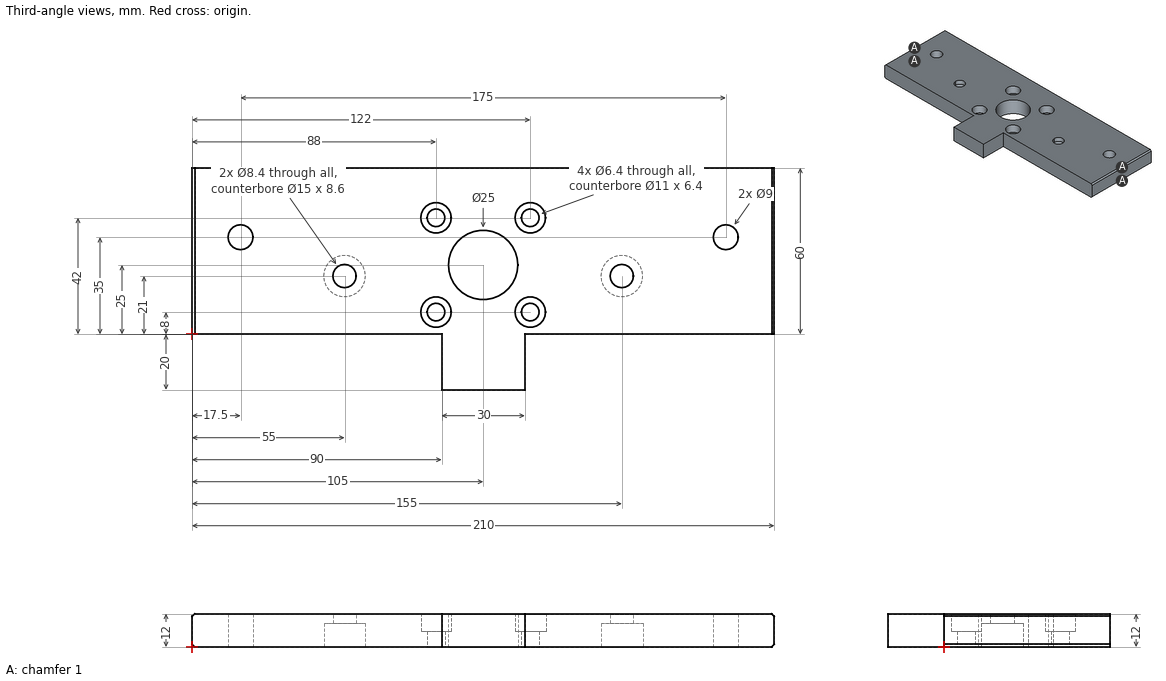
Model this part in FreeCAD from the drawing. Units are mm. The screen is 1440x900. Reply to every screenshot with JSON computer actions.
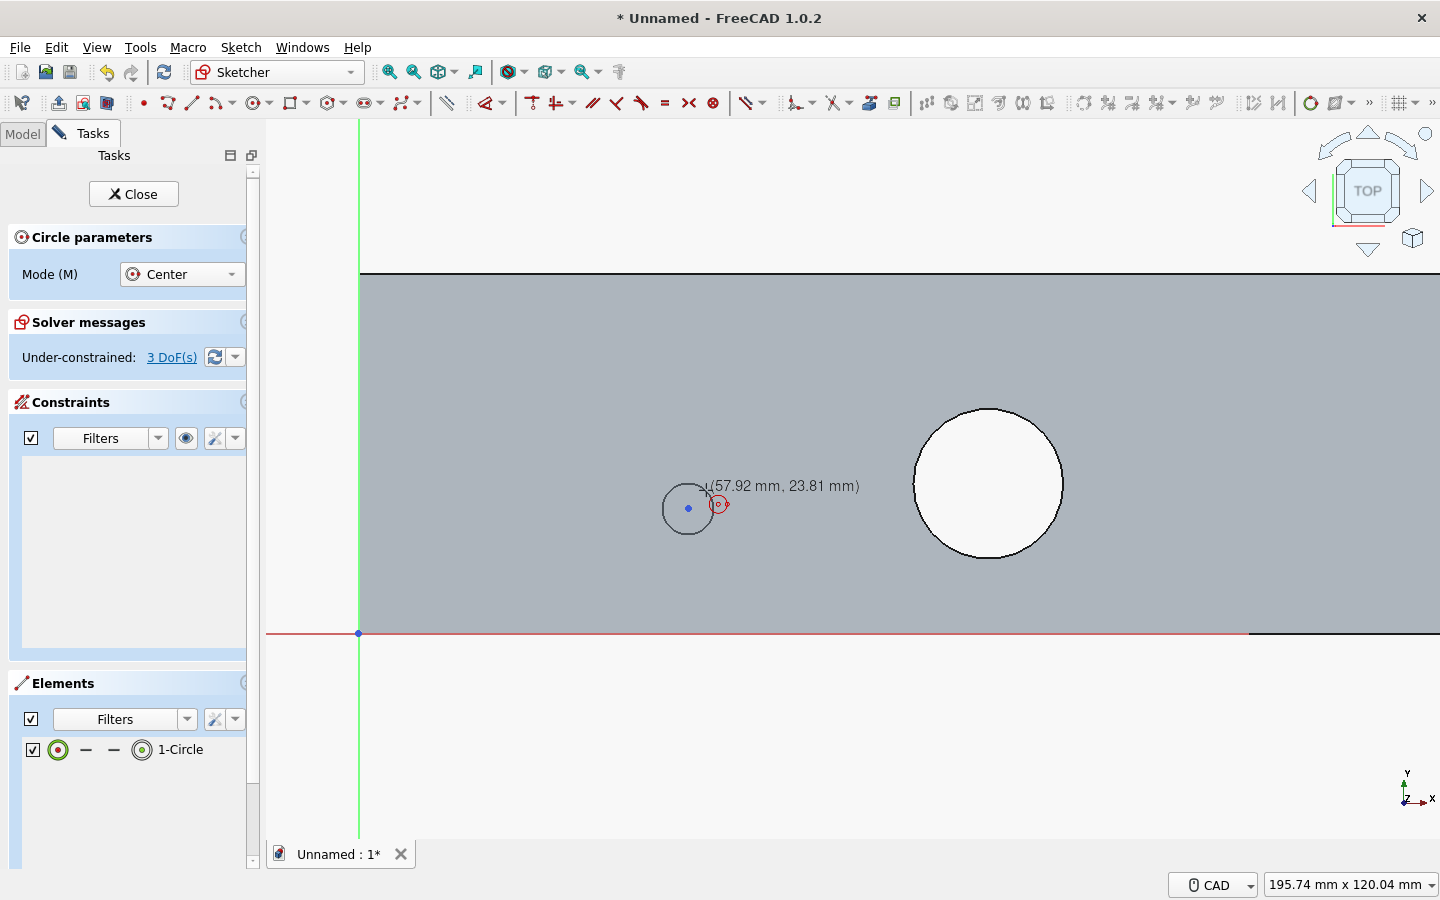
{"action": "scroll", "coordinate": [680, 318], "scroll_direction": "down", "scroll_amount": 2}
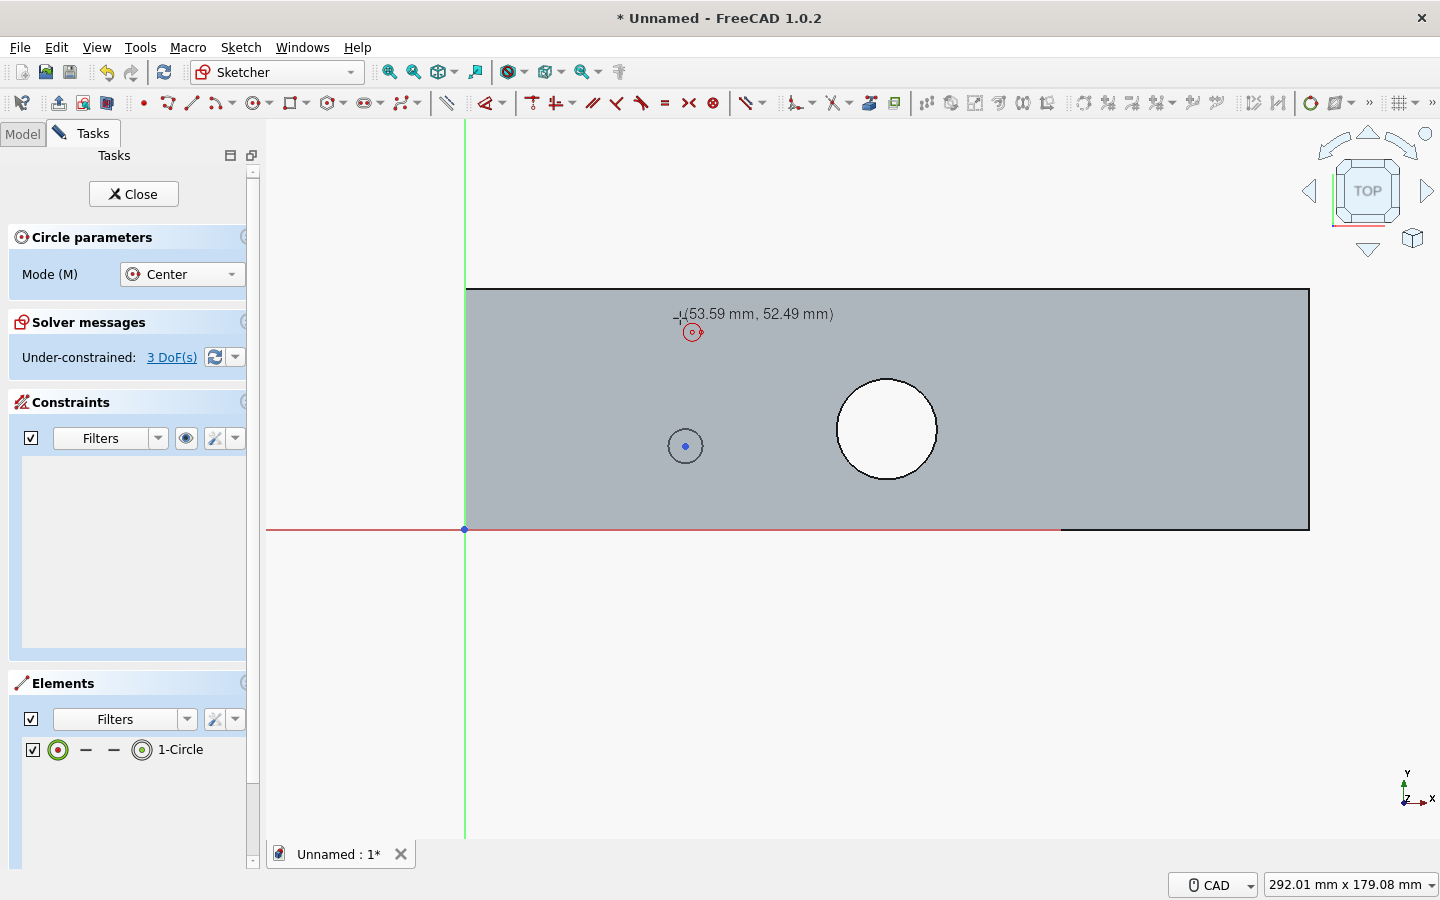
{"action": "scroll", "coordinate": [1088, 445], "scroll_direction": "up", "scroll_amount": 2}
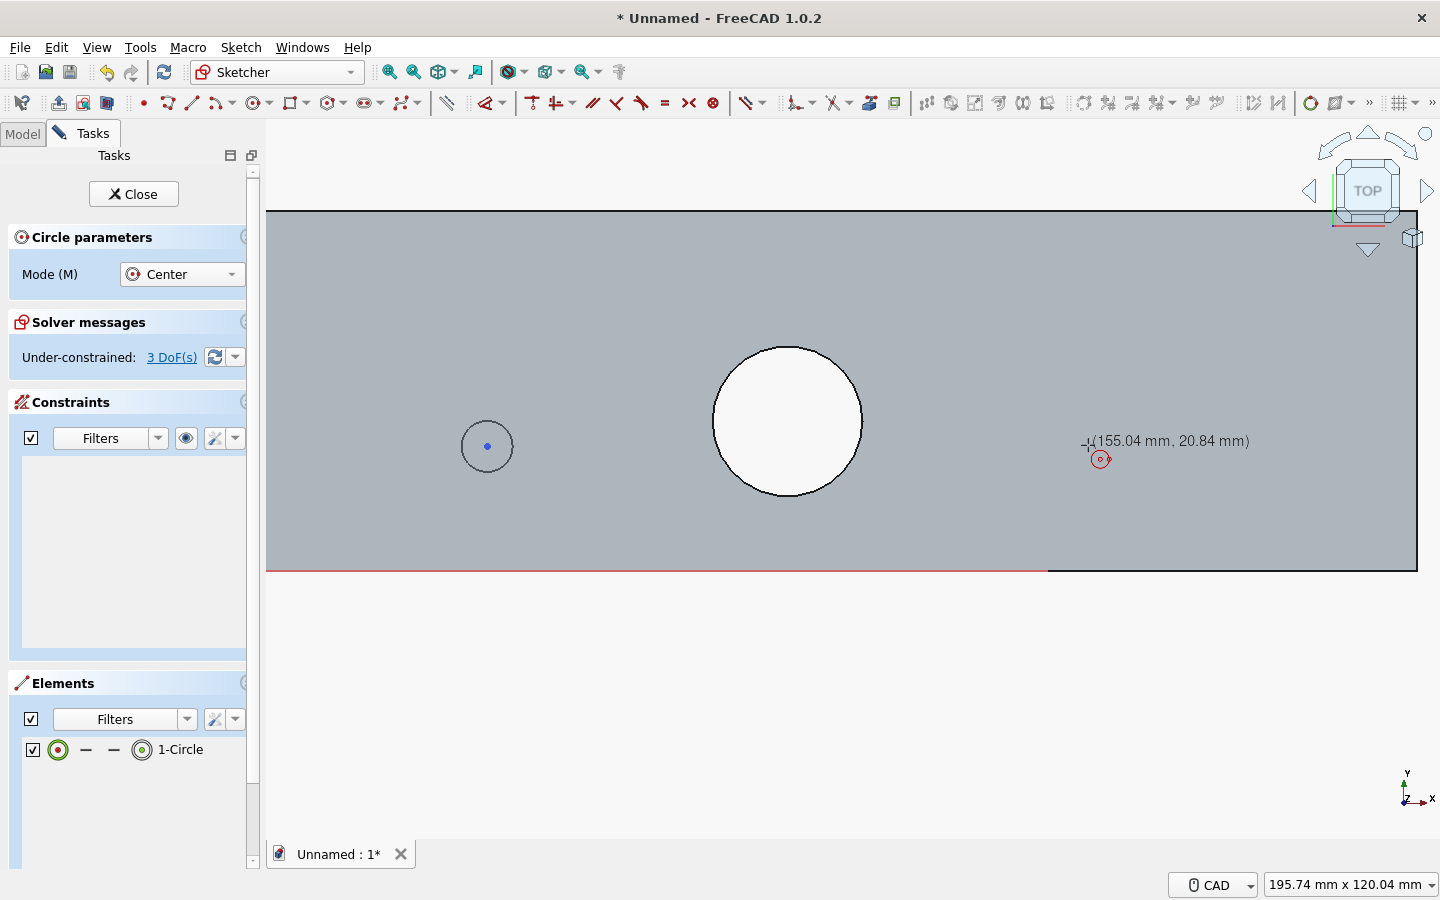
{"action": "left_click", "coordinate": [1087, 445]}
{"action": "left_click", "coordinate": [1105, 428]}
{"action": "key", "text": "Escape"}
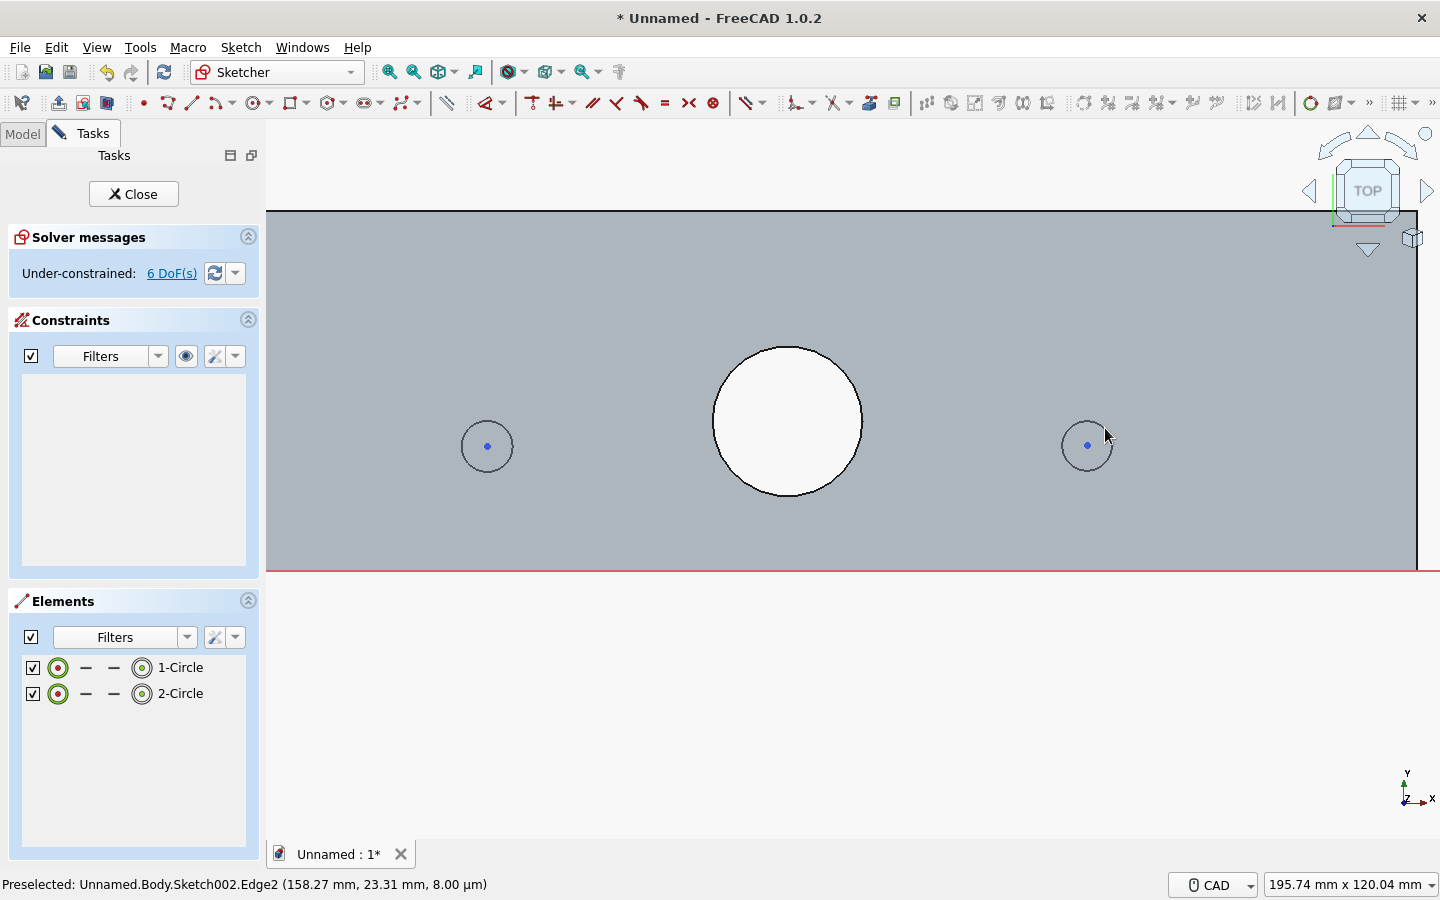
{"action": "left_click", "coordinate": [505, 428]}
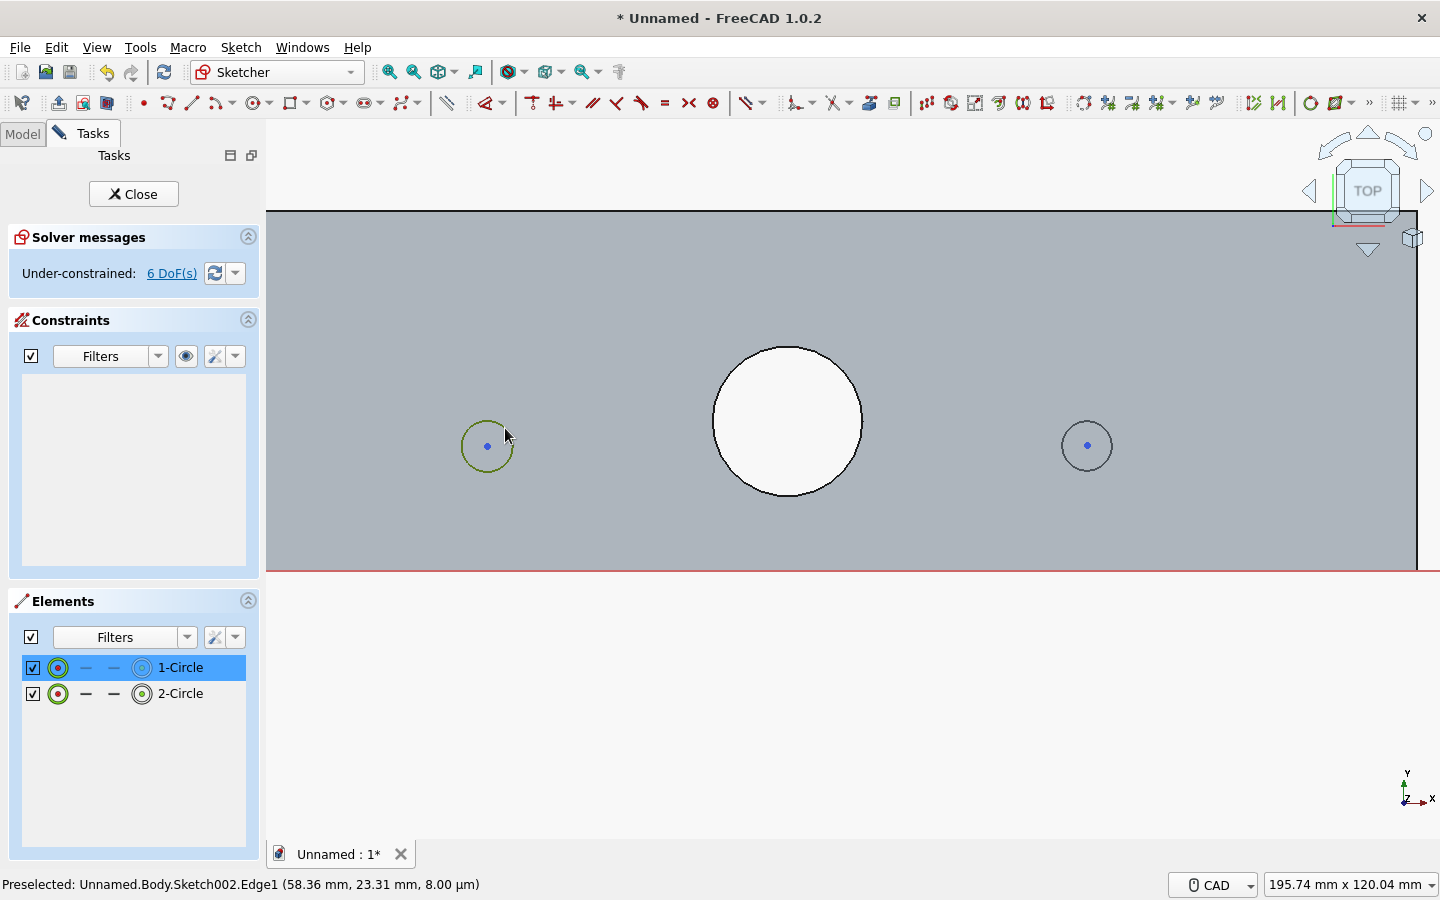
{"action": "left_click", "coordinate": [1104, 428]}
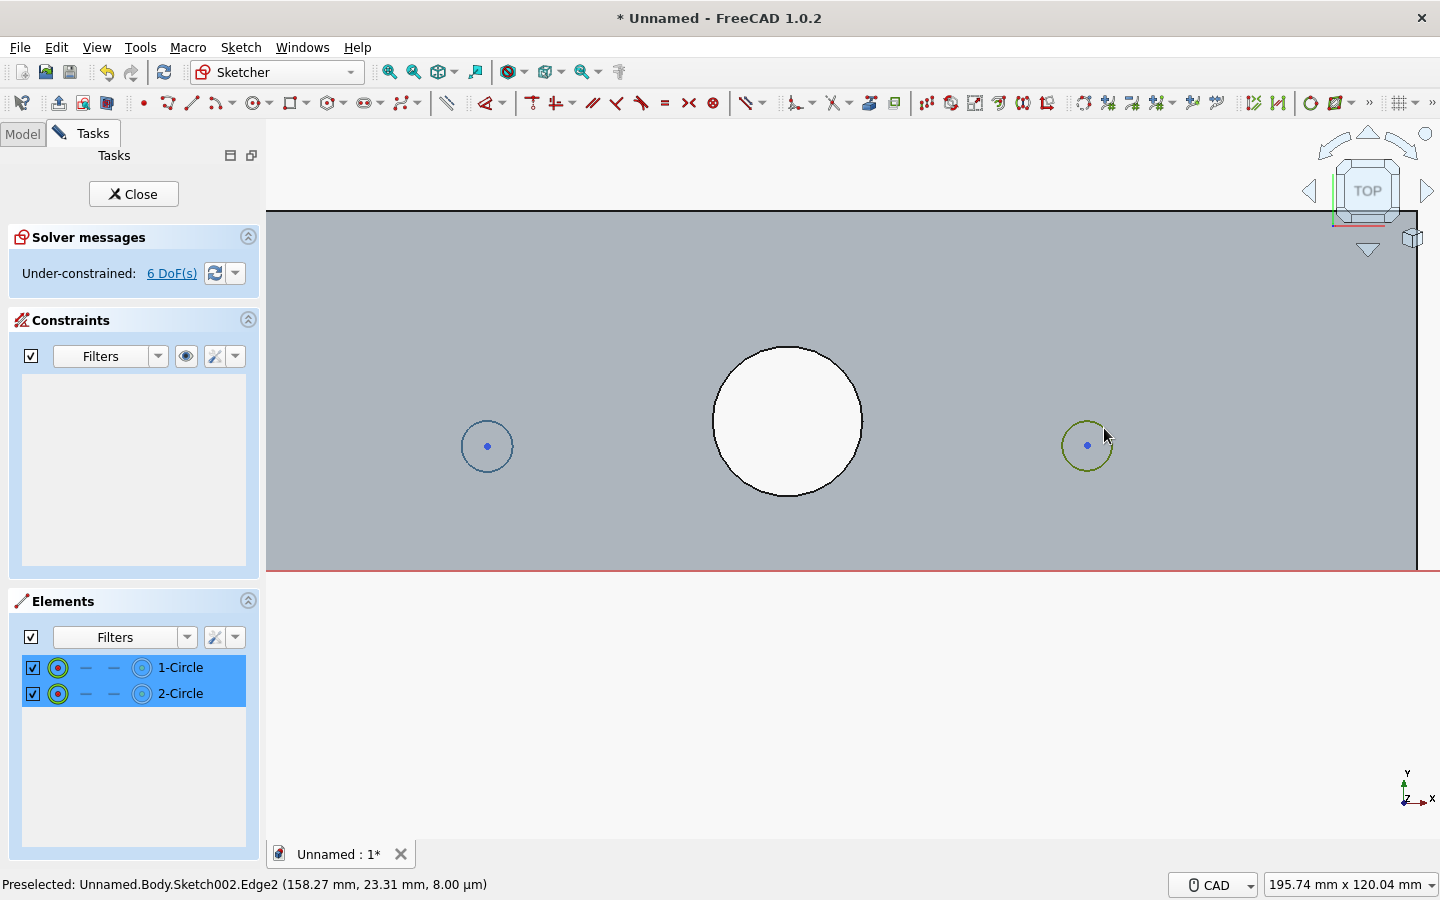
{"action": "left_click", "coordinate": [666, 104]}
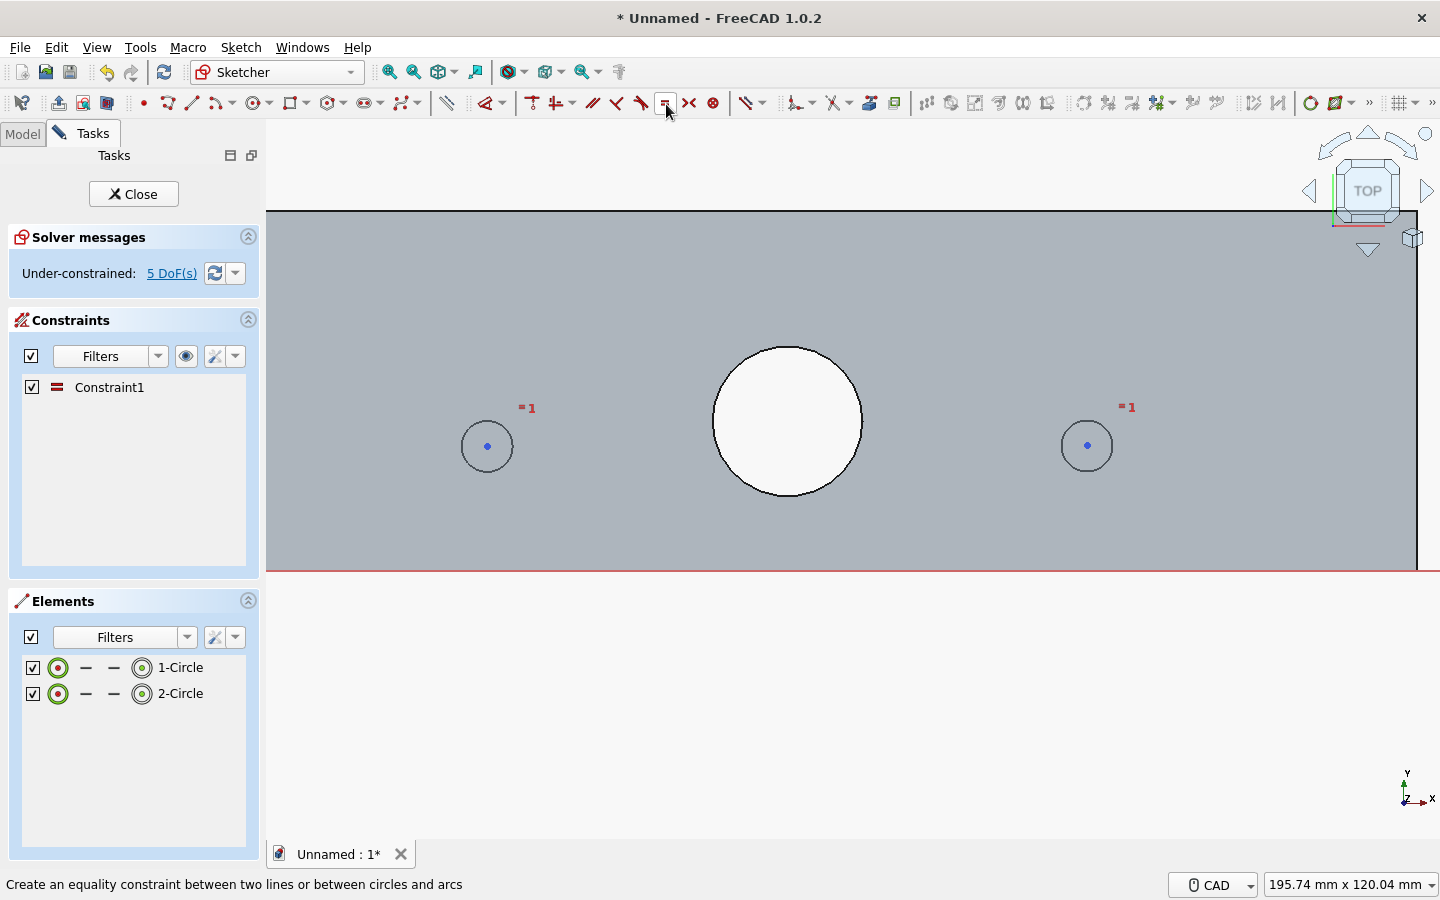
{"action": "left_click", "coordinate": [487, 446]}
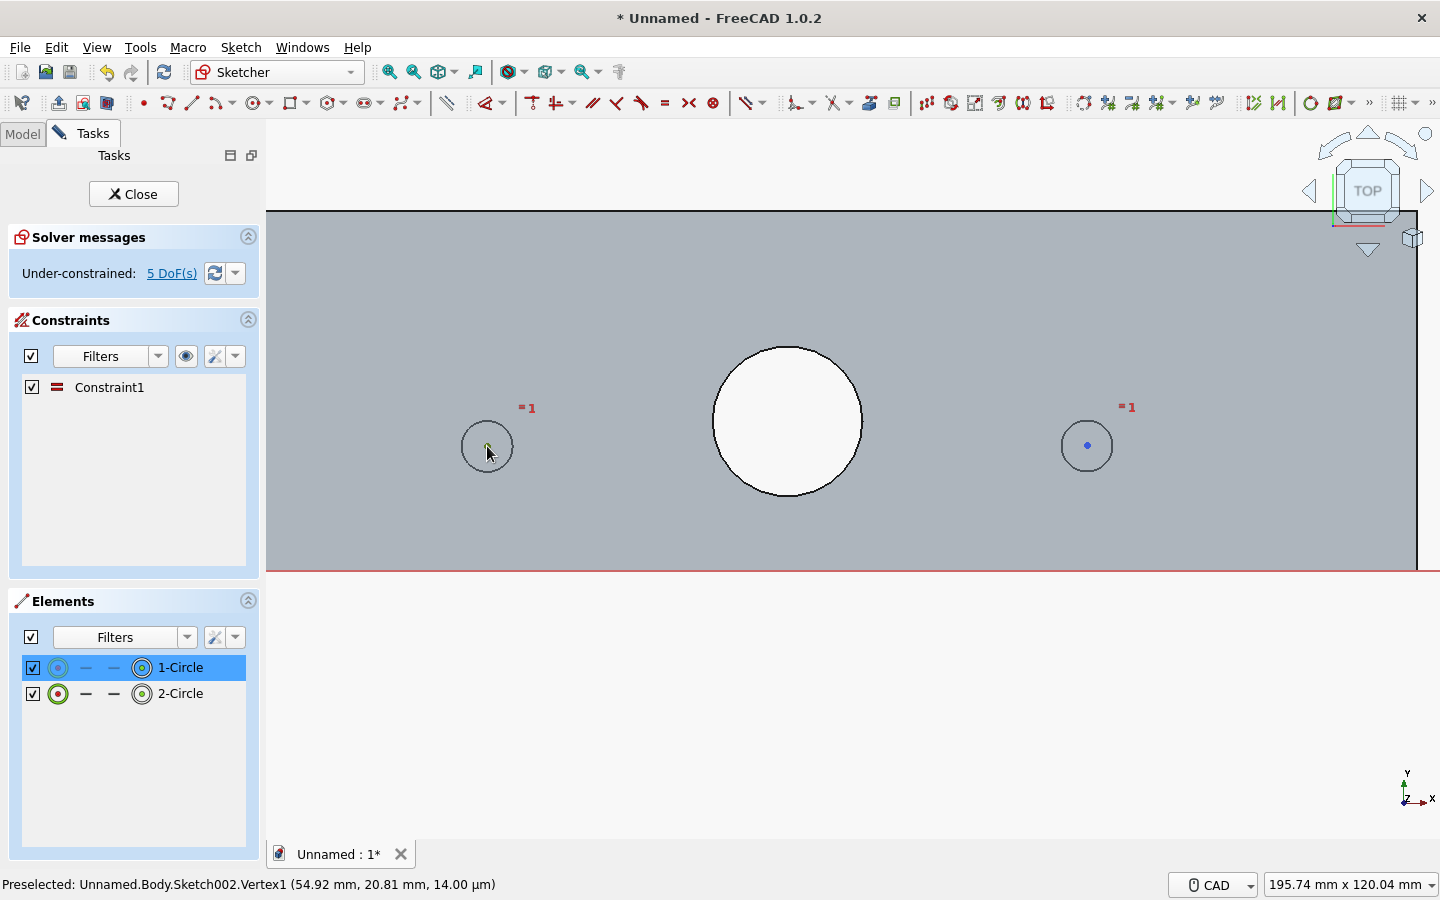
{"action": "left_click", "coordinate": [1087, 446]}